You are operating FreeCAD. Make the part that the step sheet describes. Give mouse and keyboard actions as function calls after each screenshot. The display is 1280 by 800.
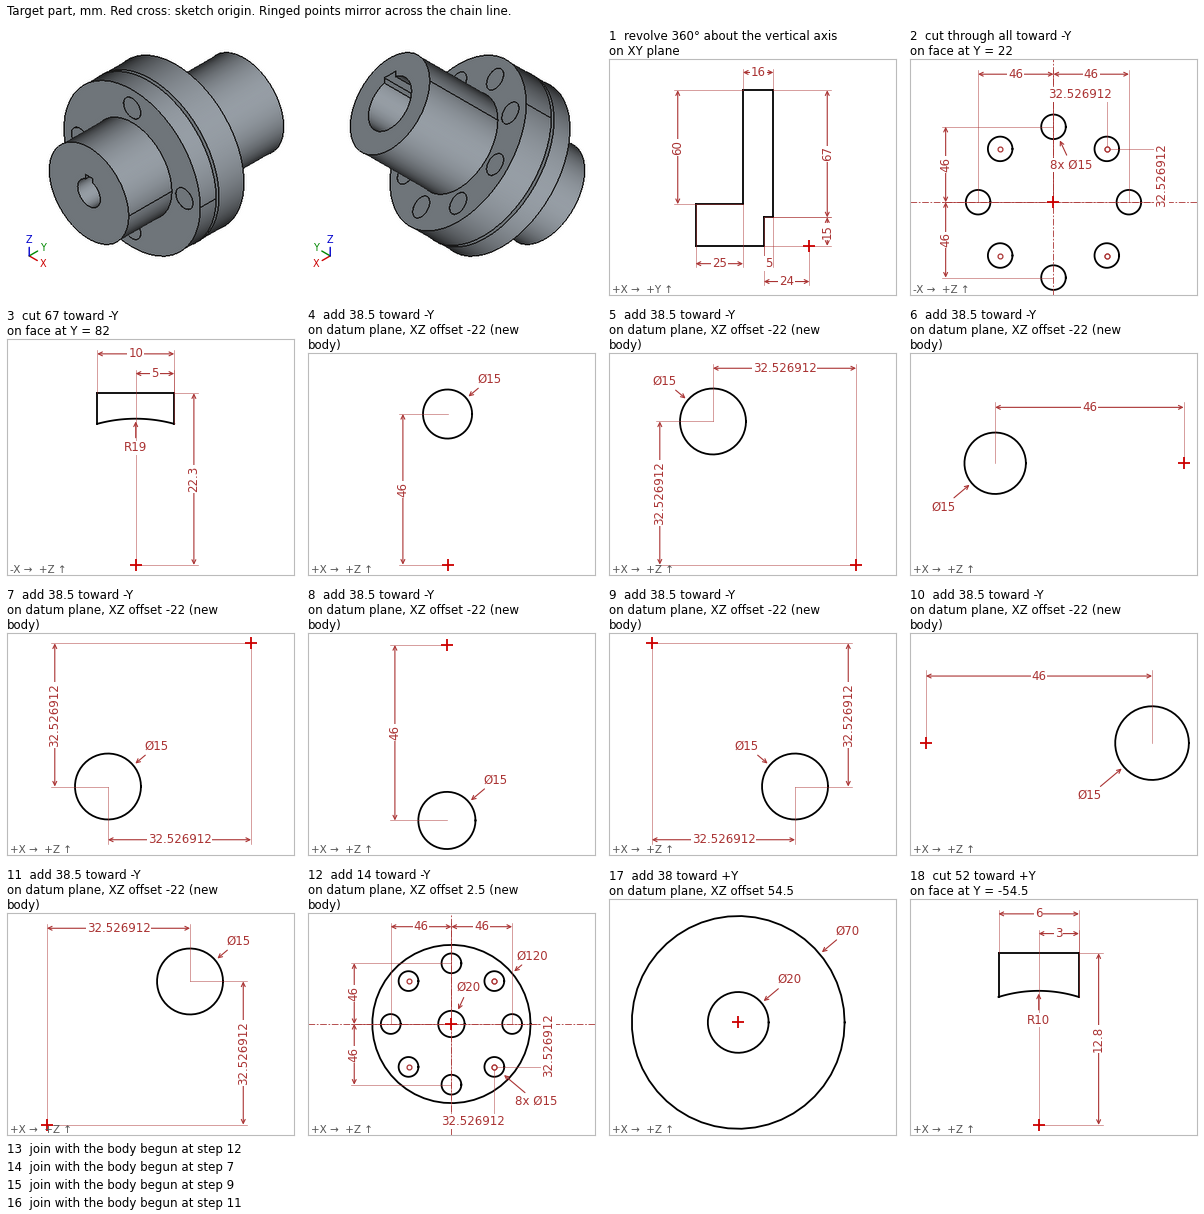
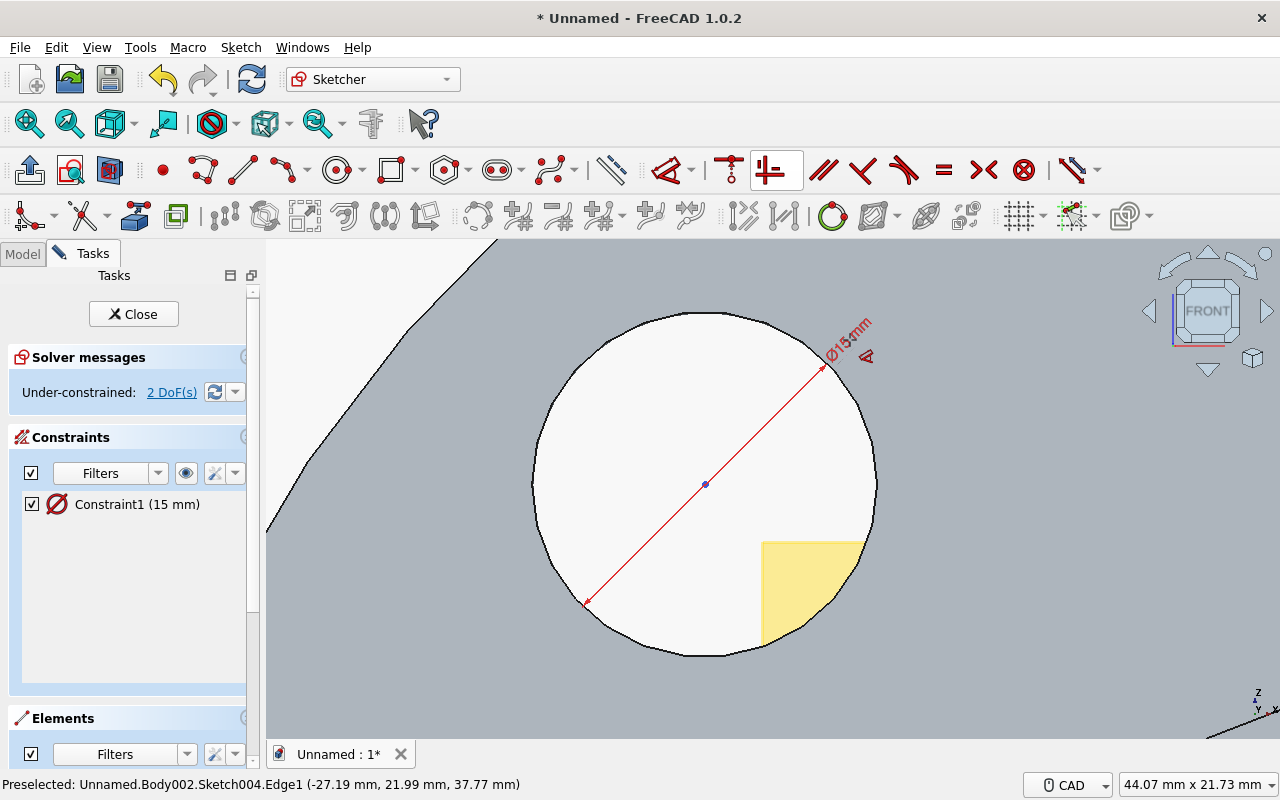
click(705, 485)
click(910, 451)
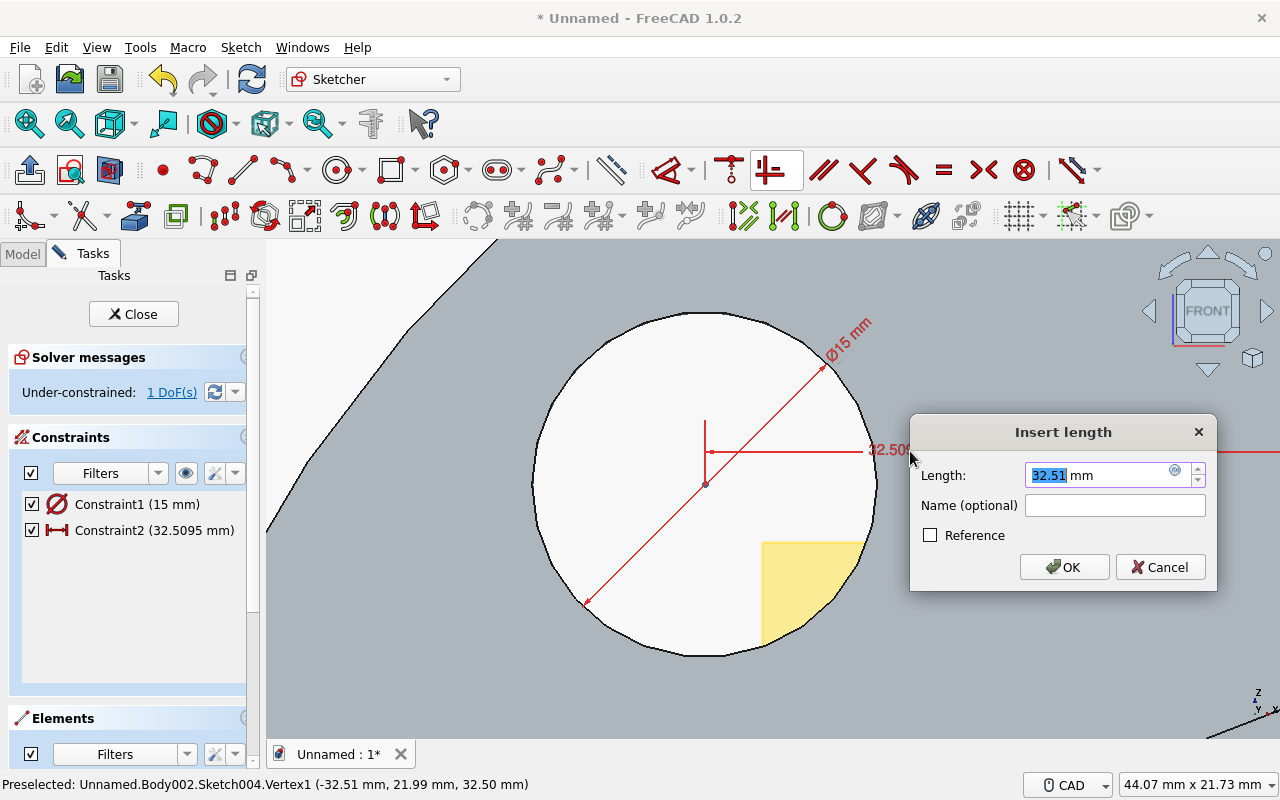
text(32.526912)
key(Return)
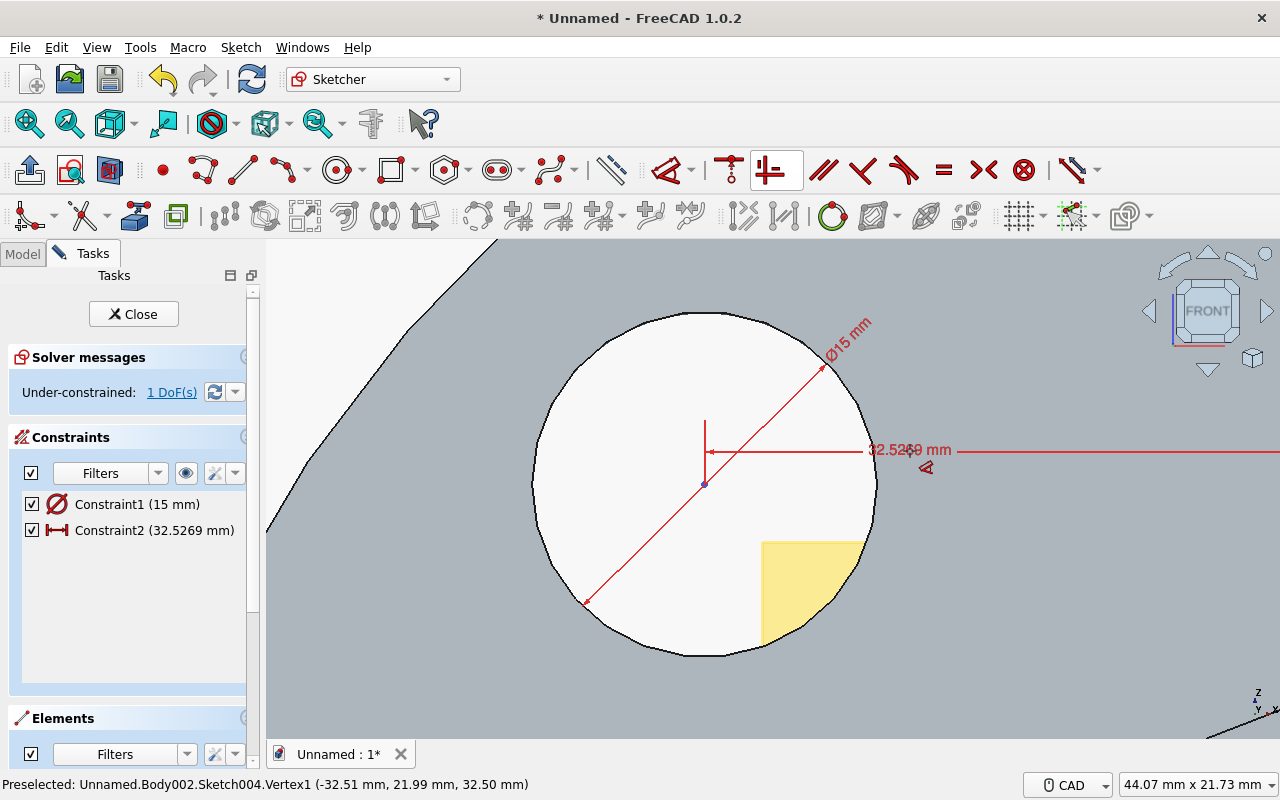
click(705, 485)
click(671, 598)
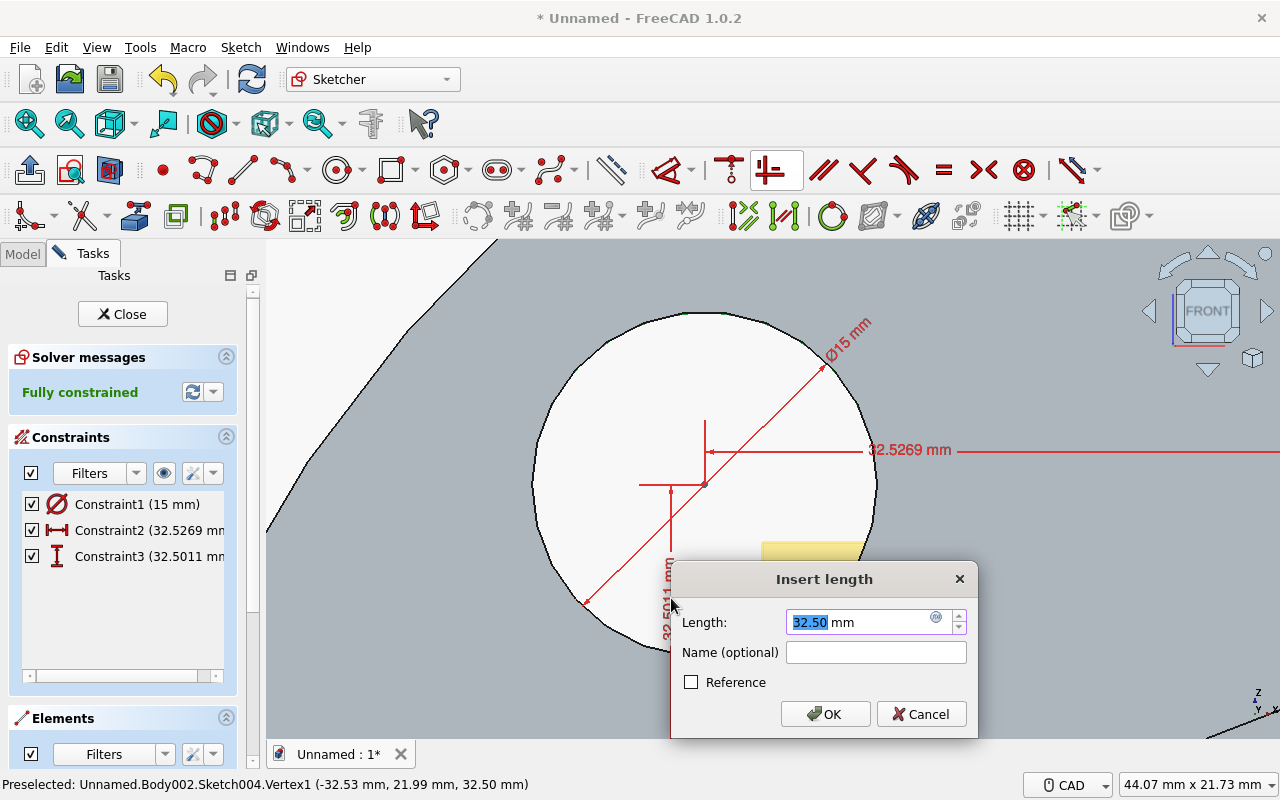
text(32.526912)
key(Return)
key(Escape)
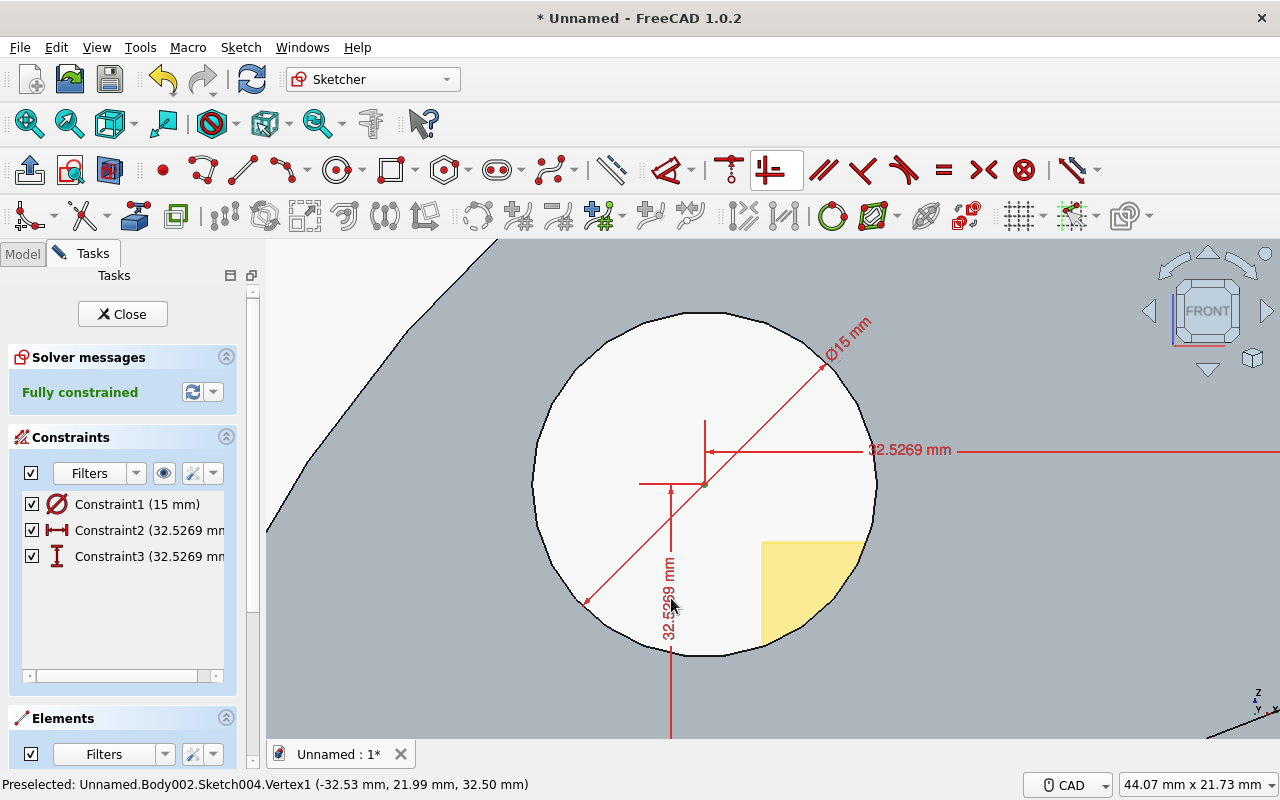
click(123, 314)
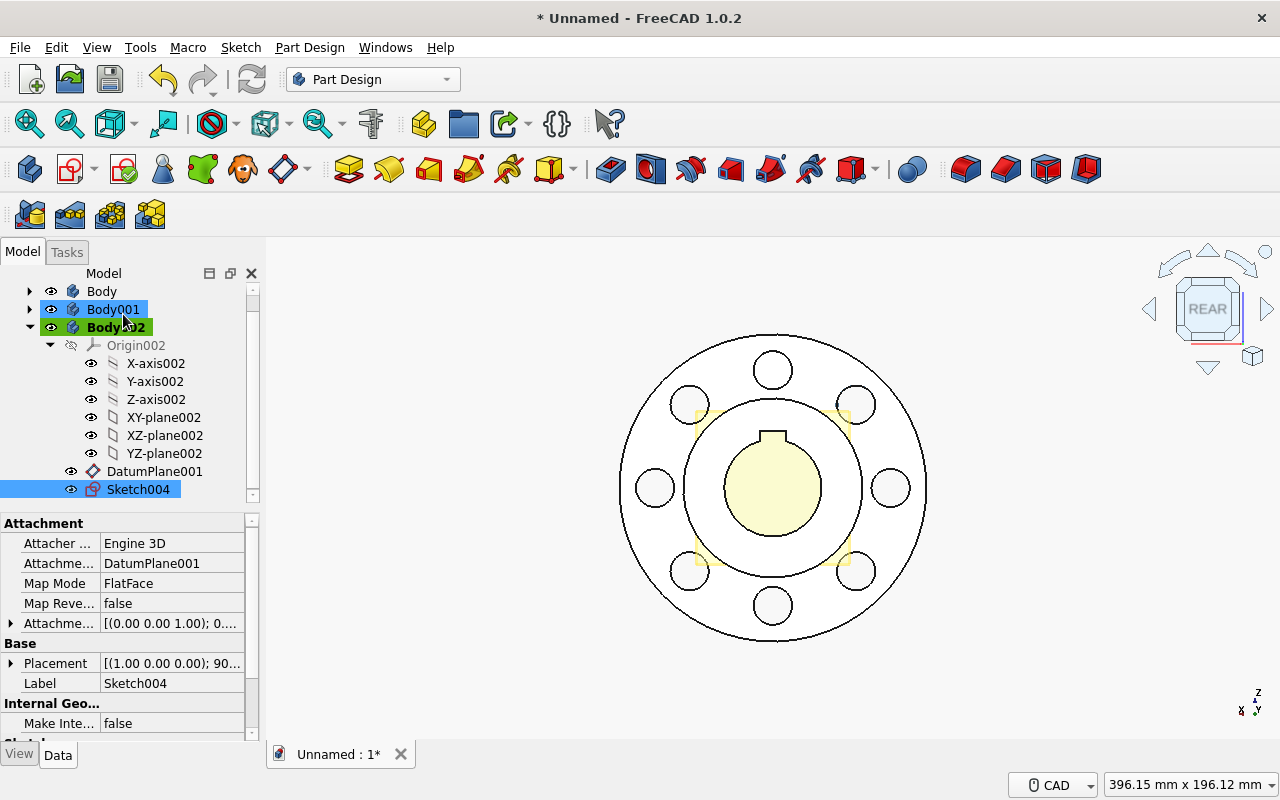
click(350, 170)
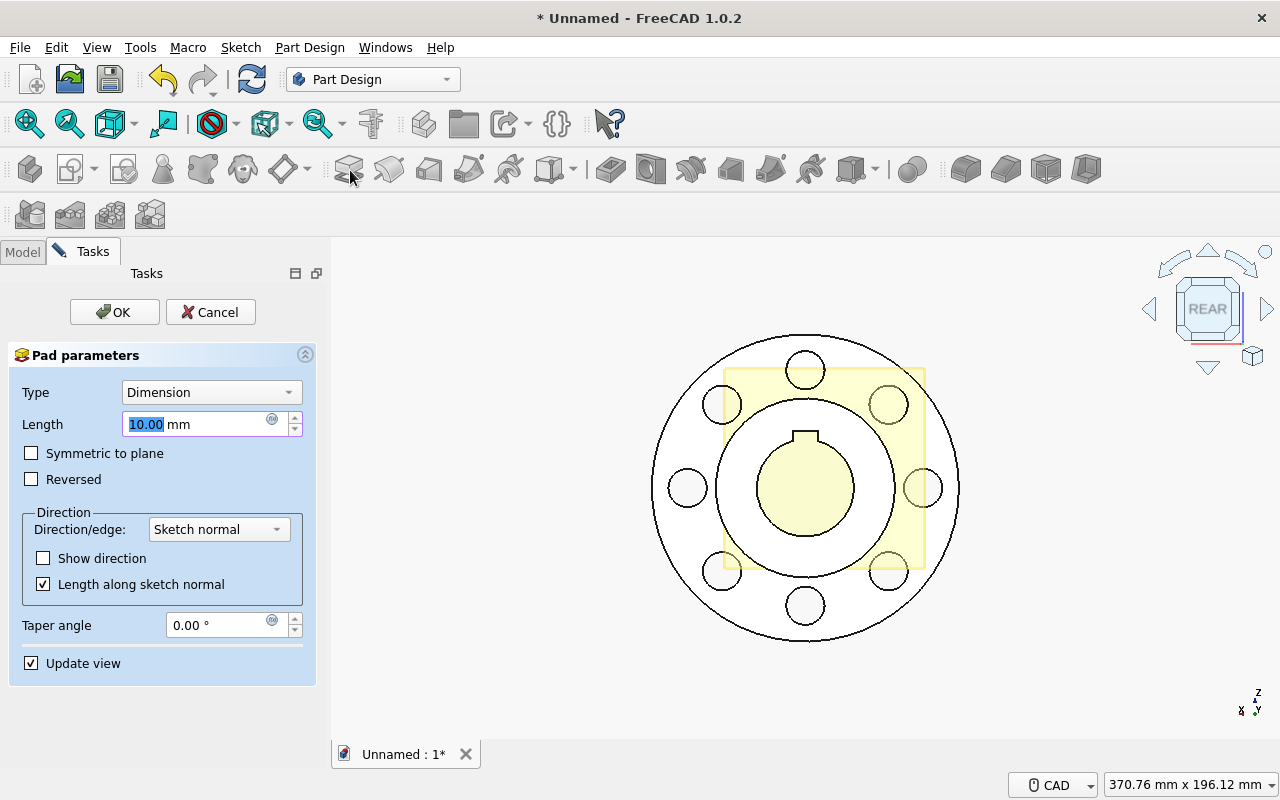
text(38.5)
key(Tab)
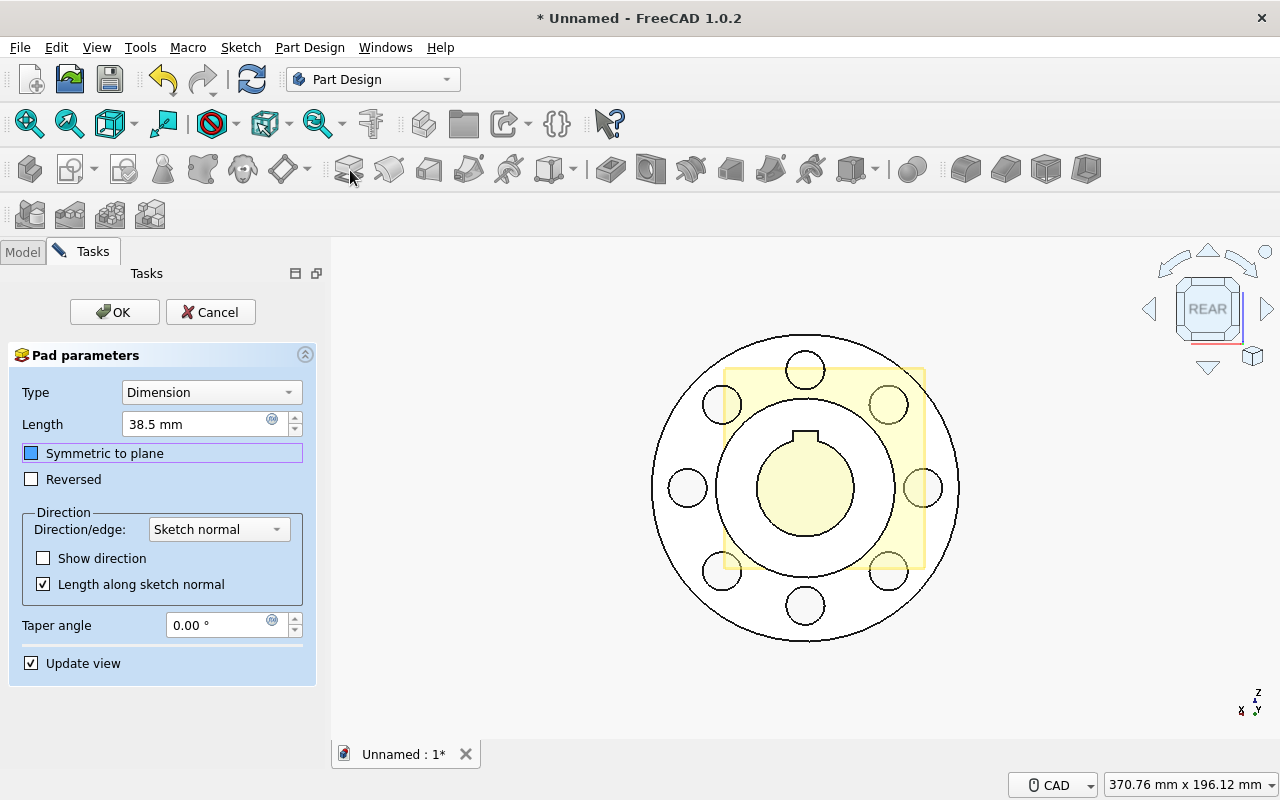
click(115, 312)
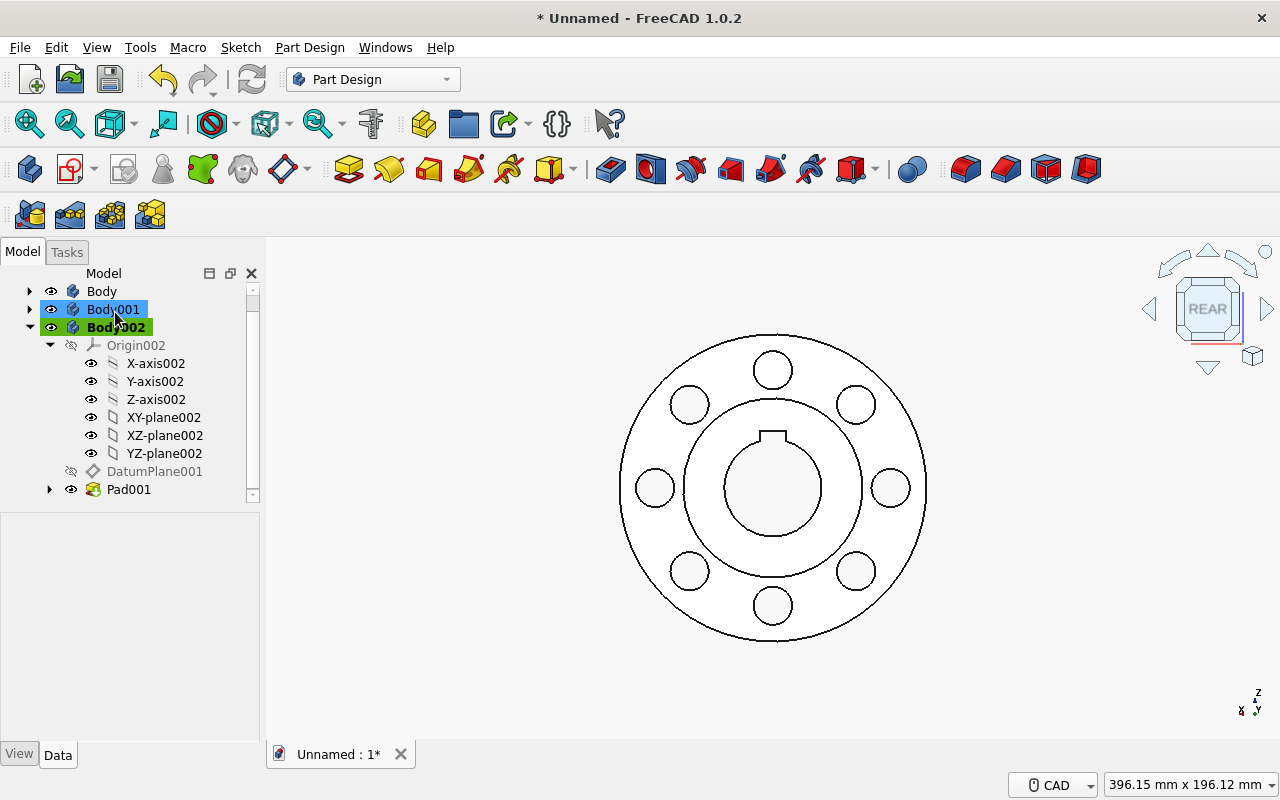
click(30, 124)